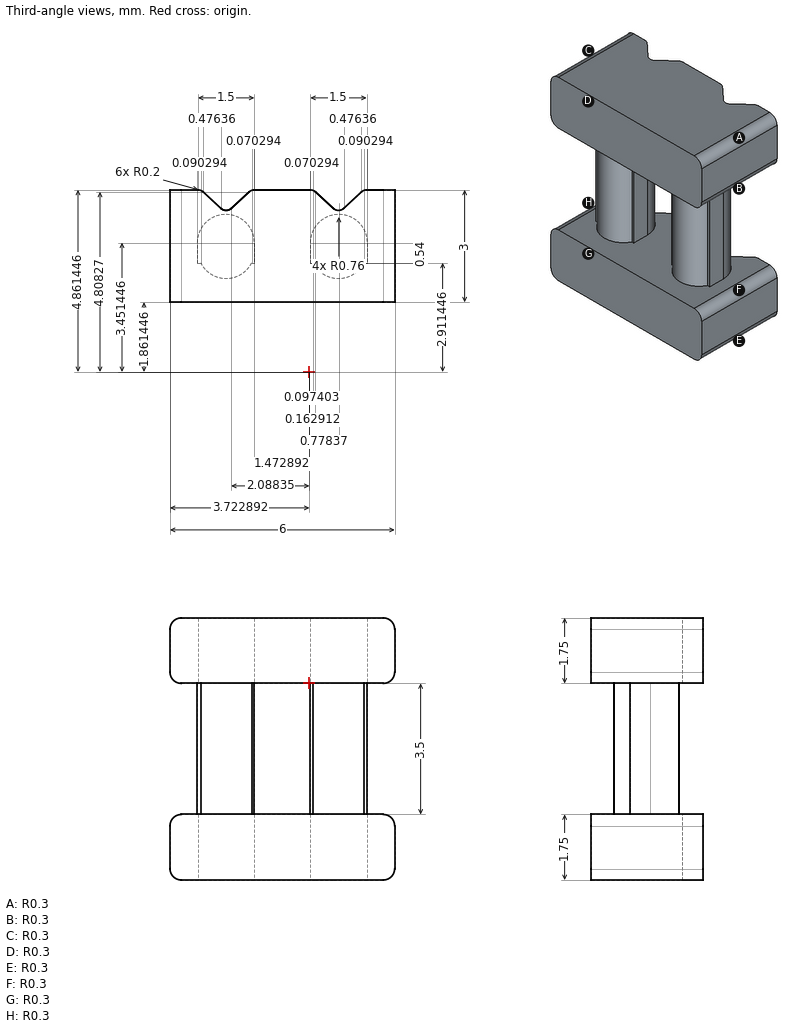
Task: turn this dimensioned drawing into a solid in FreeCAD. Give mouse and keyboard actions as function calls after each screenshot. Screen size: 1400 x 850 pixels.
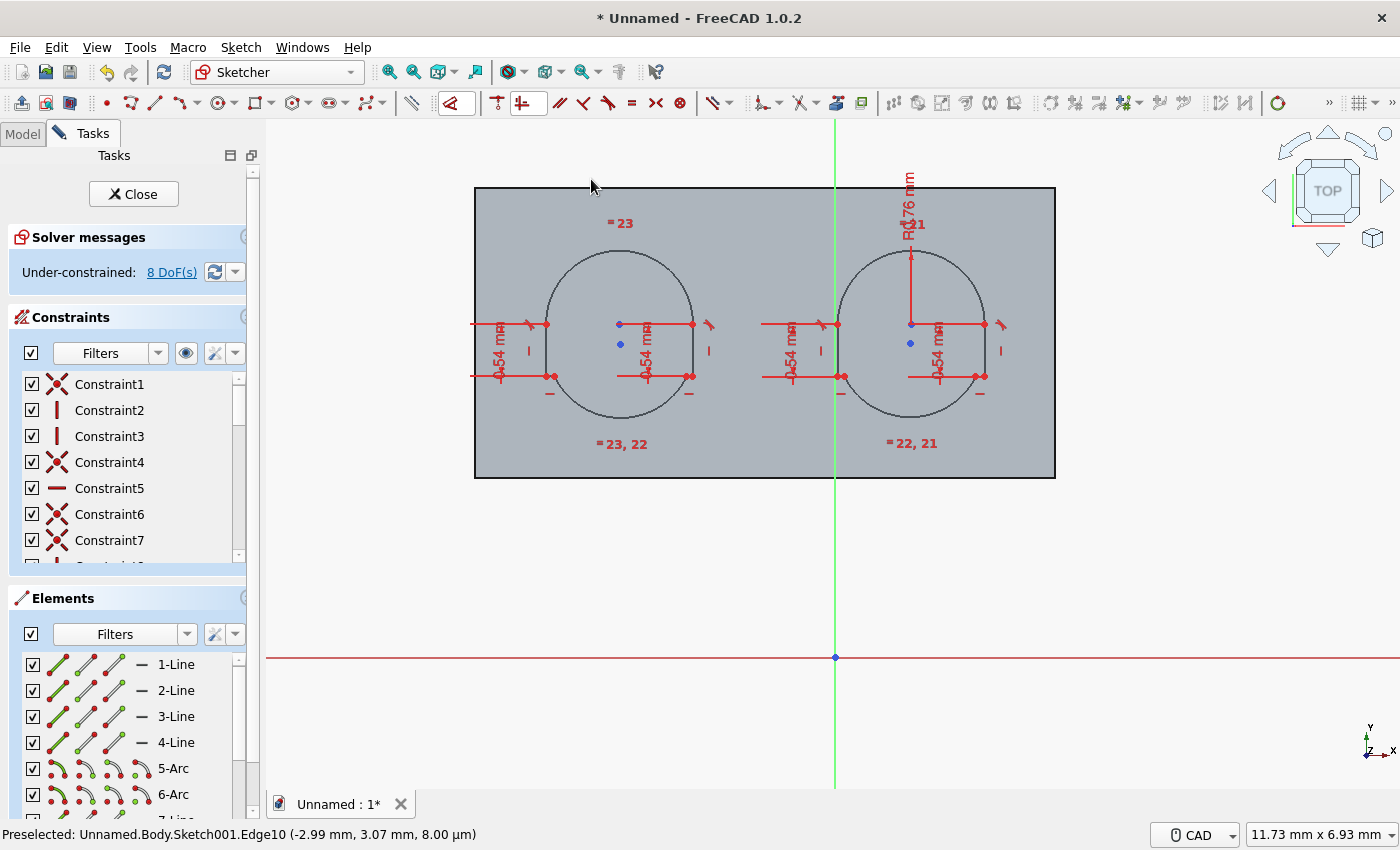
scroll(841, 377, up, 9)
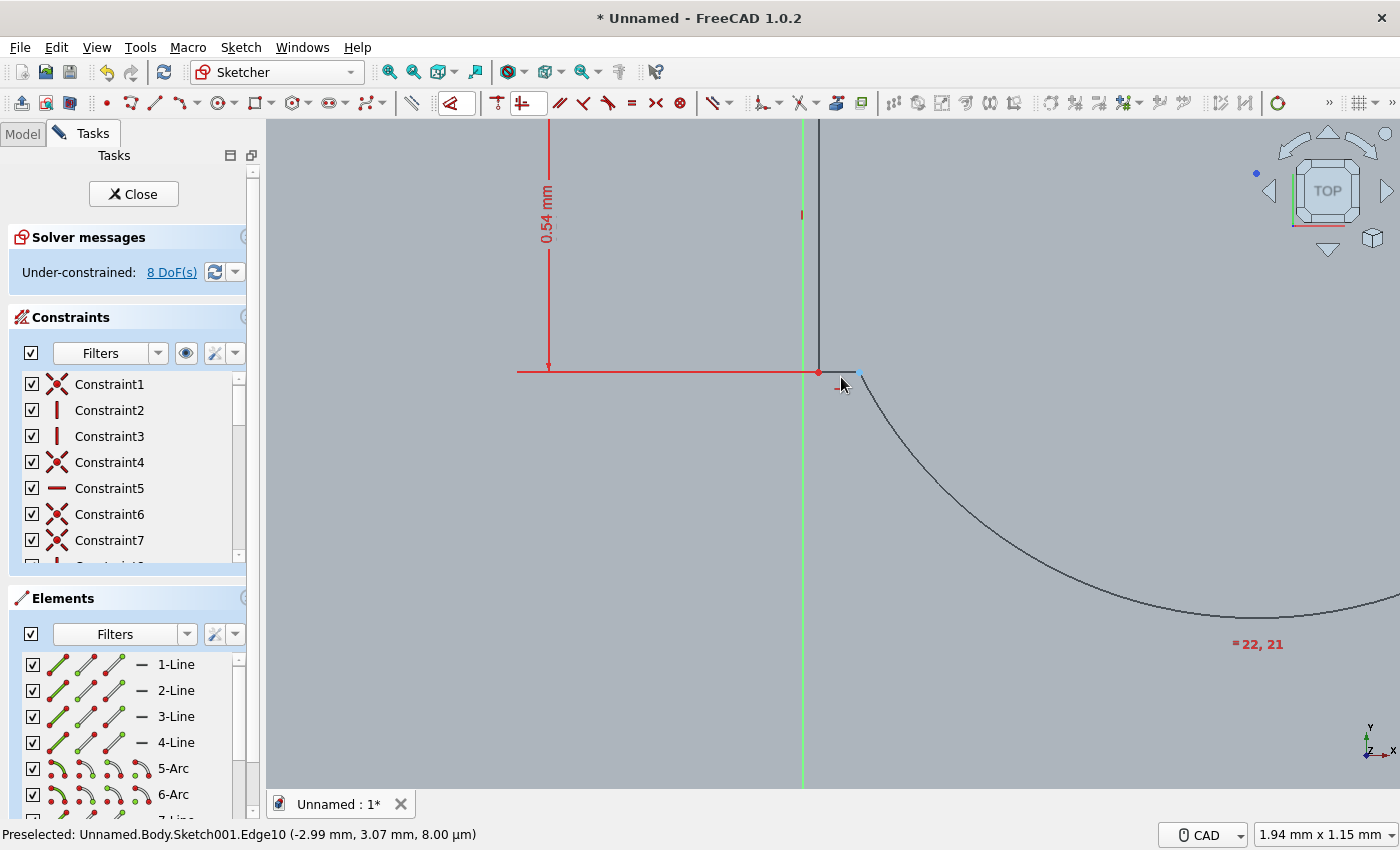
click(839, 372)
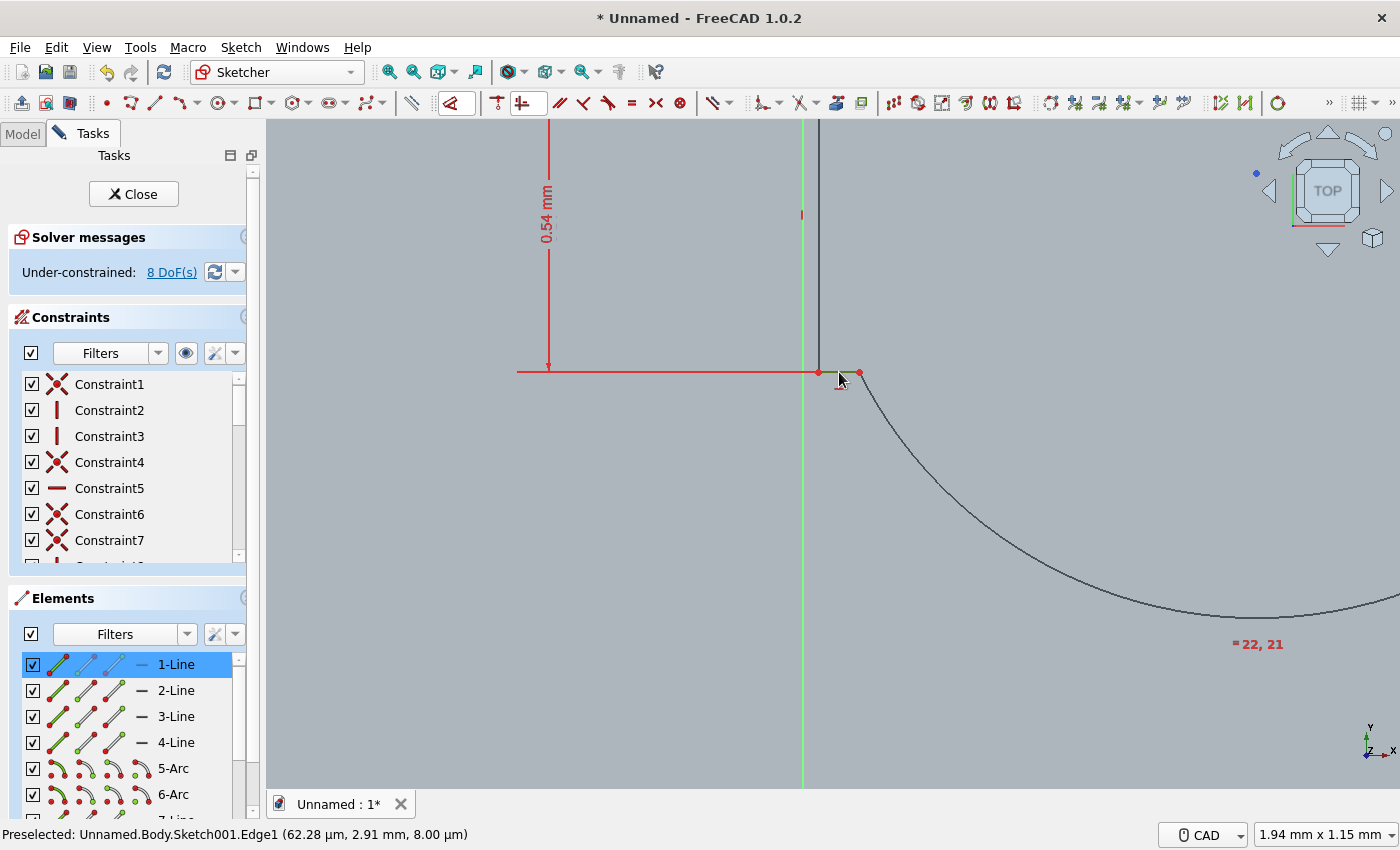
click(470, 104)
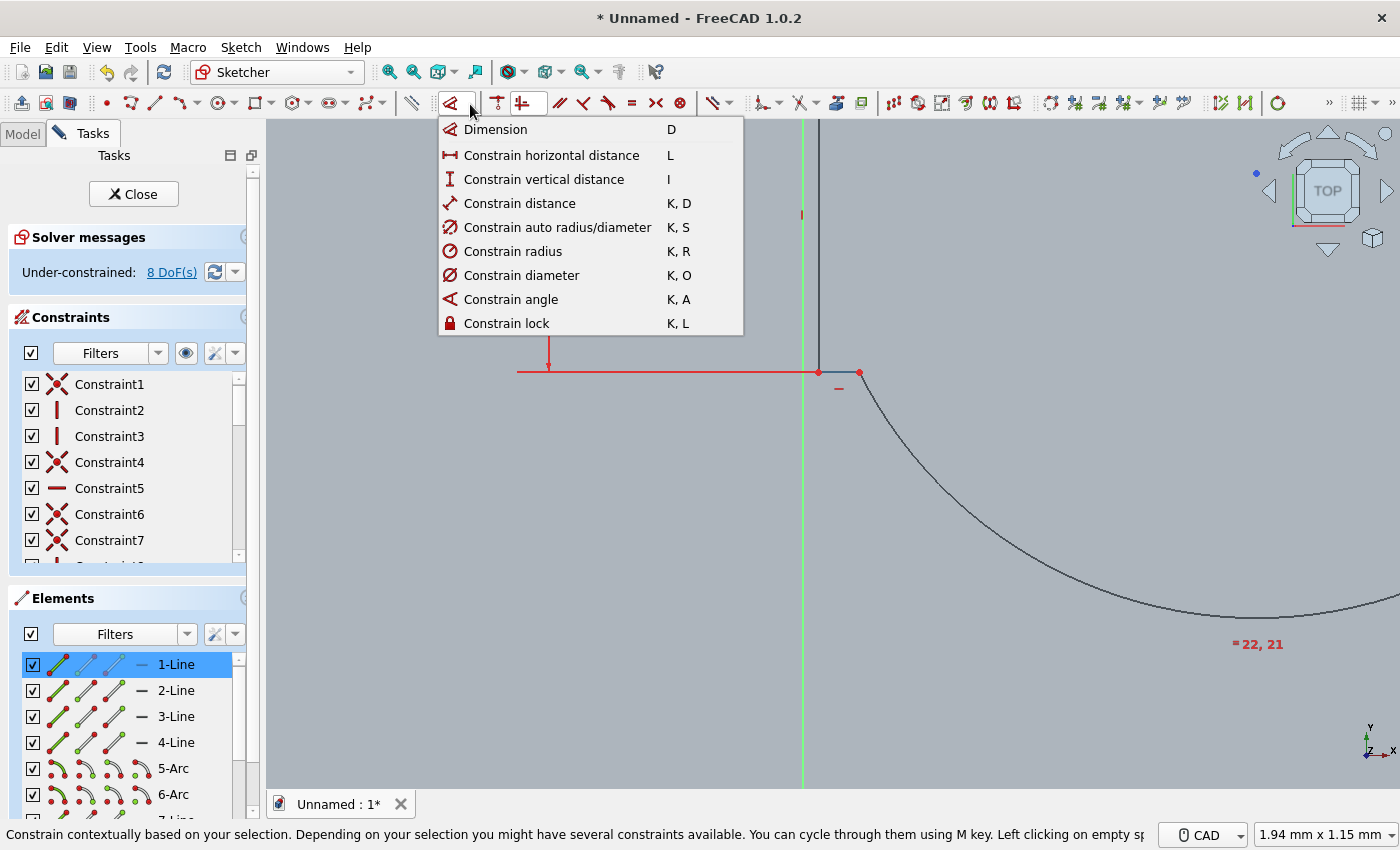
click(591, 155)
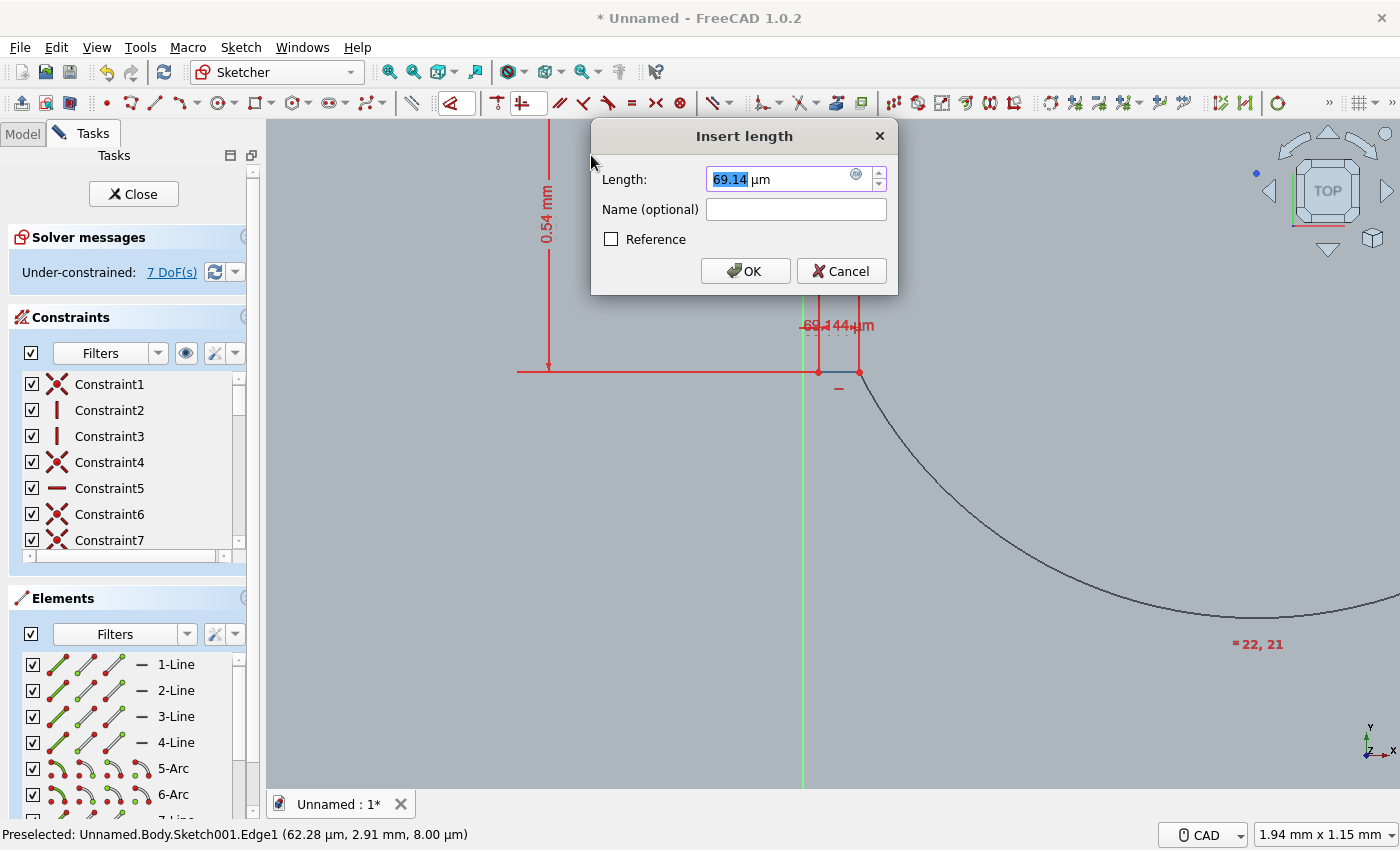
key(ctrl+a)
text(0.070294 mm)
key(Return)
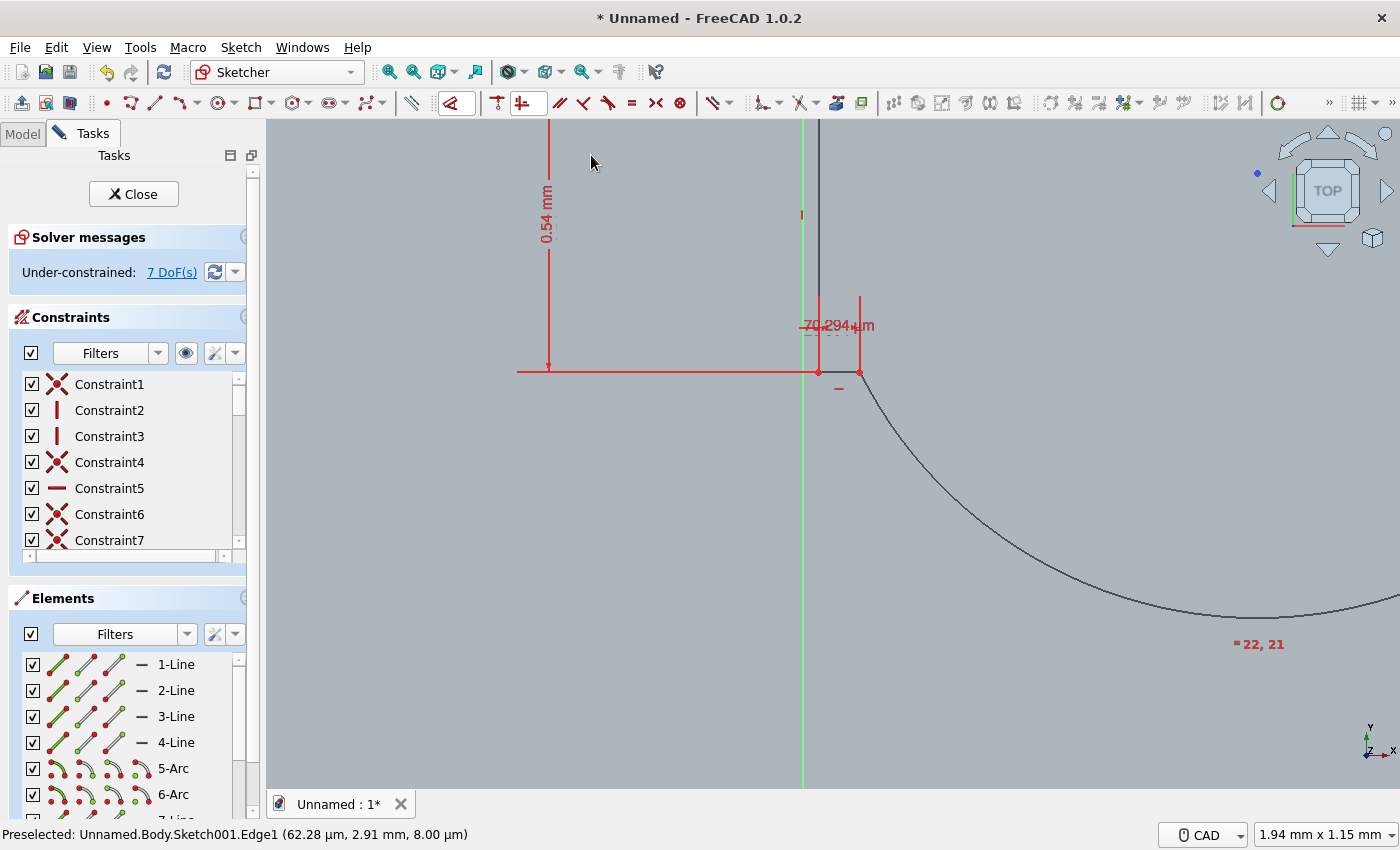
scroll(841, 377, down, 9)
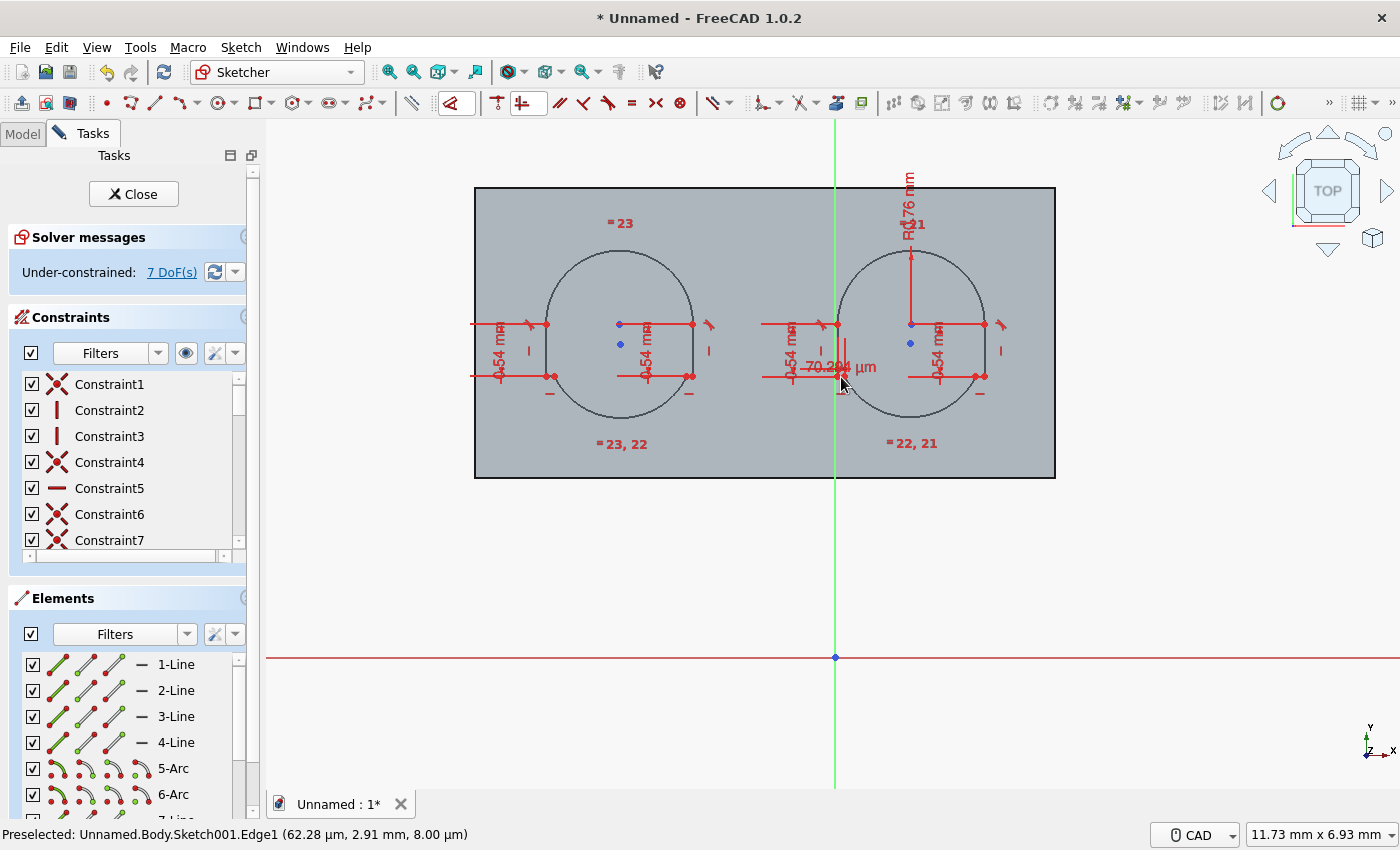
scroll(982, 377, up, 9)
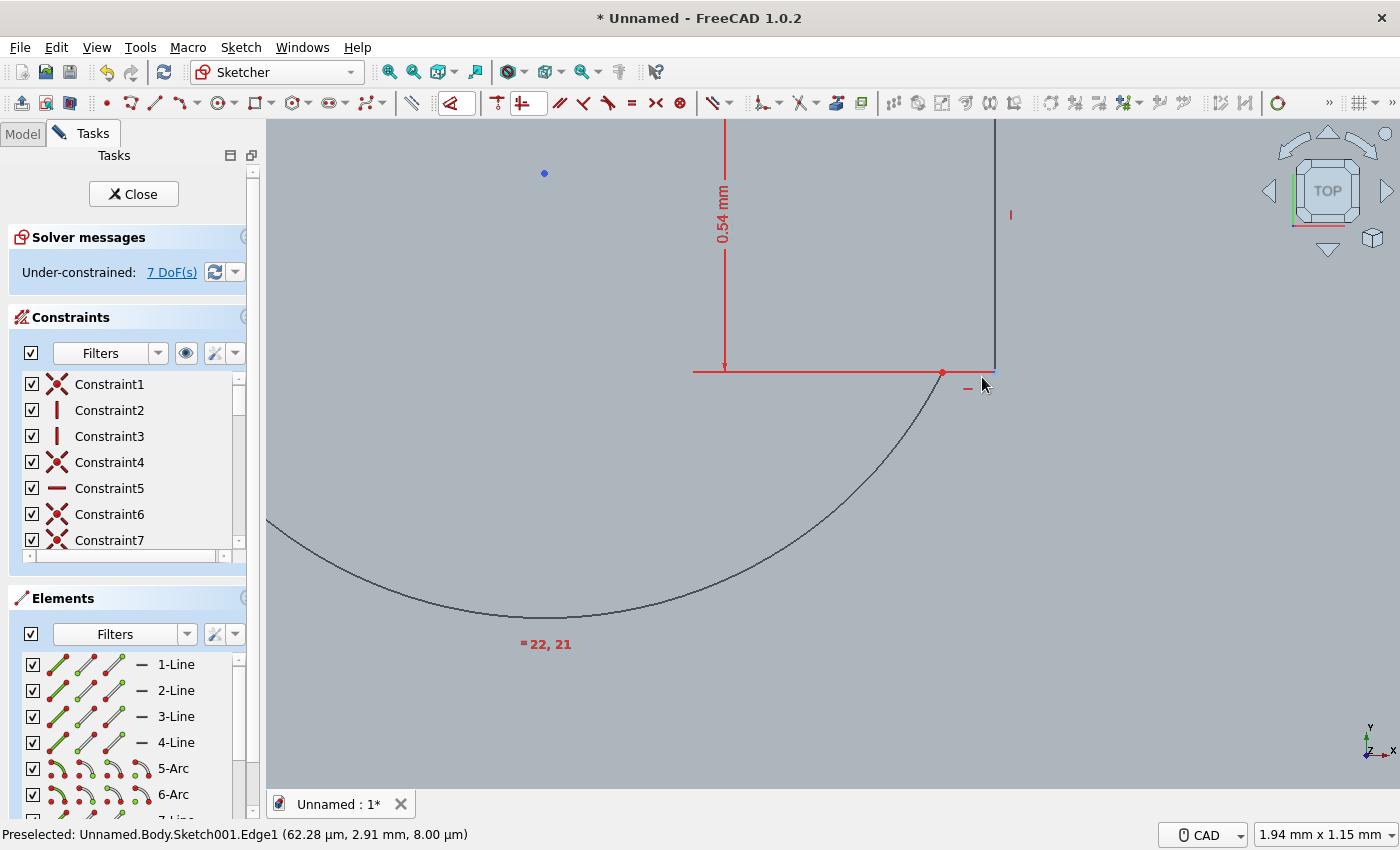
click(979, 372)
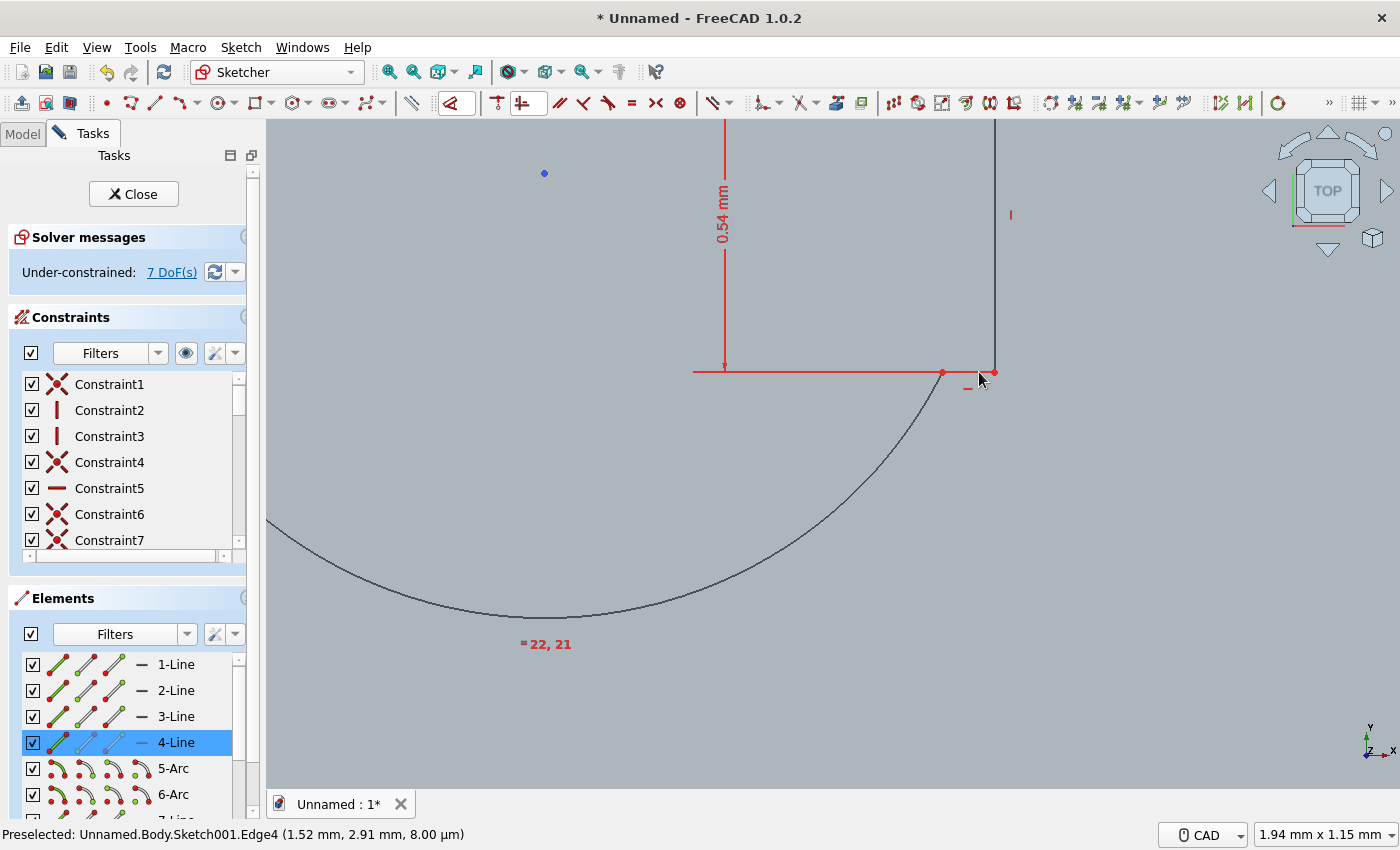
key(l)